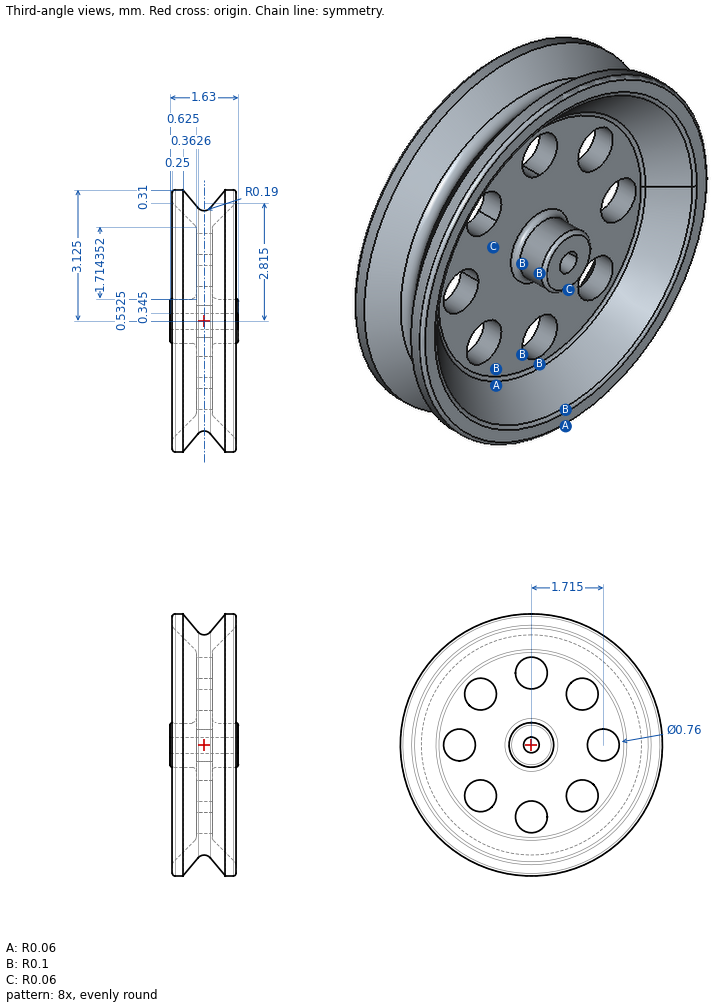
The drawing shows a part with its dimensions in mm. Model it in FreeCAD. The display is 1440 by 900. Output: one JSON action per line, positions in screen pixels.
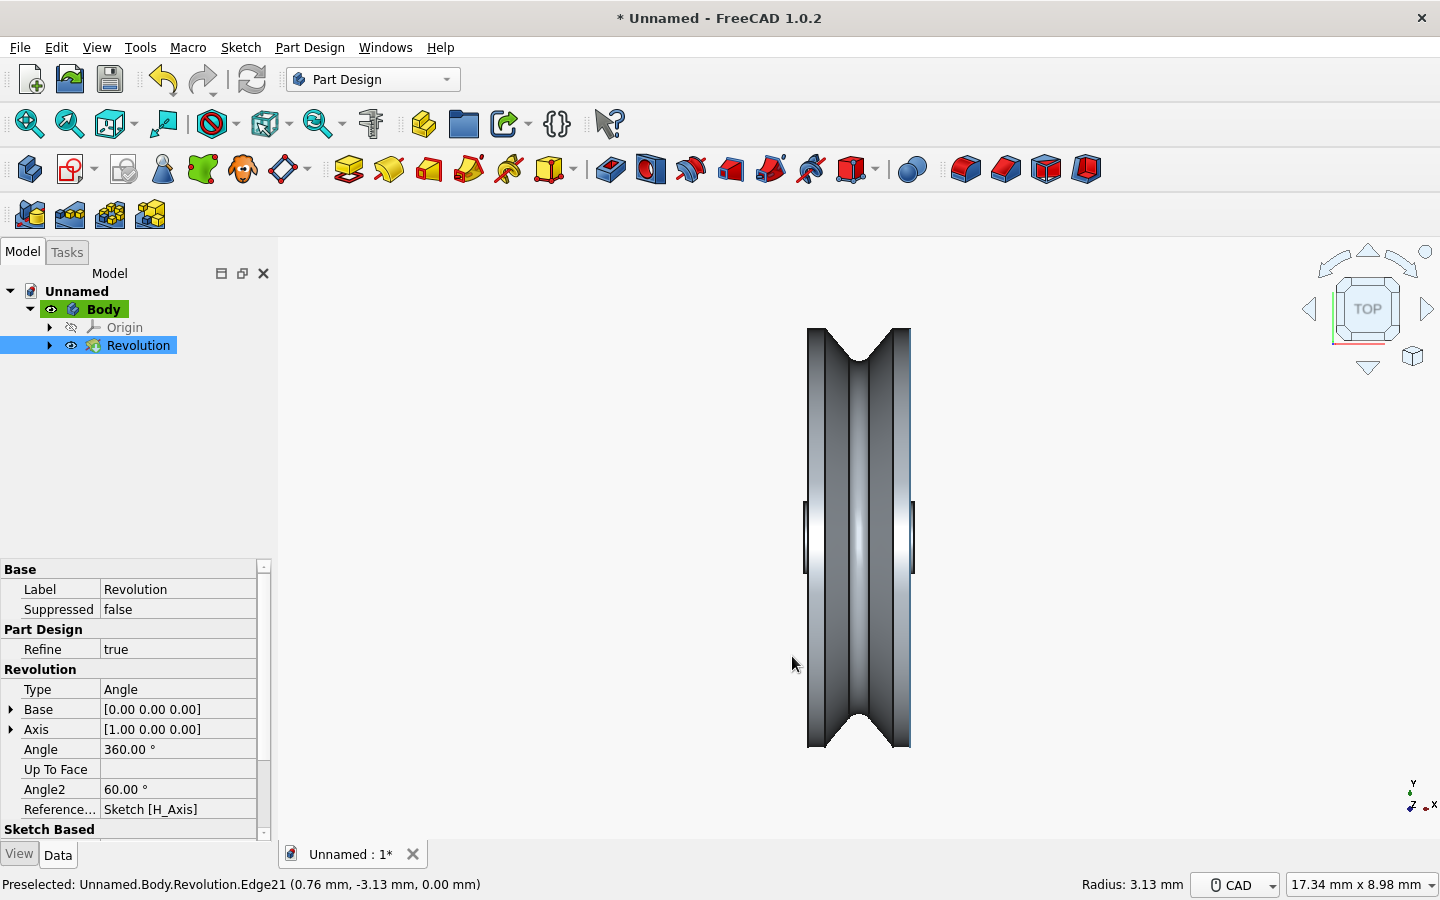
{"action": "left_click", "coordinate": [808, 706], "text": "ctrl"}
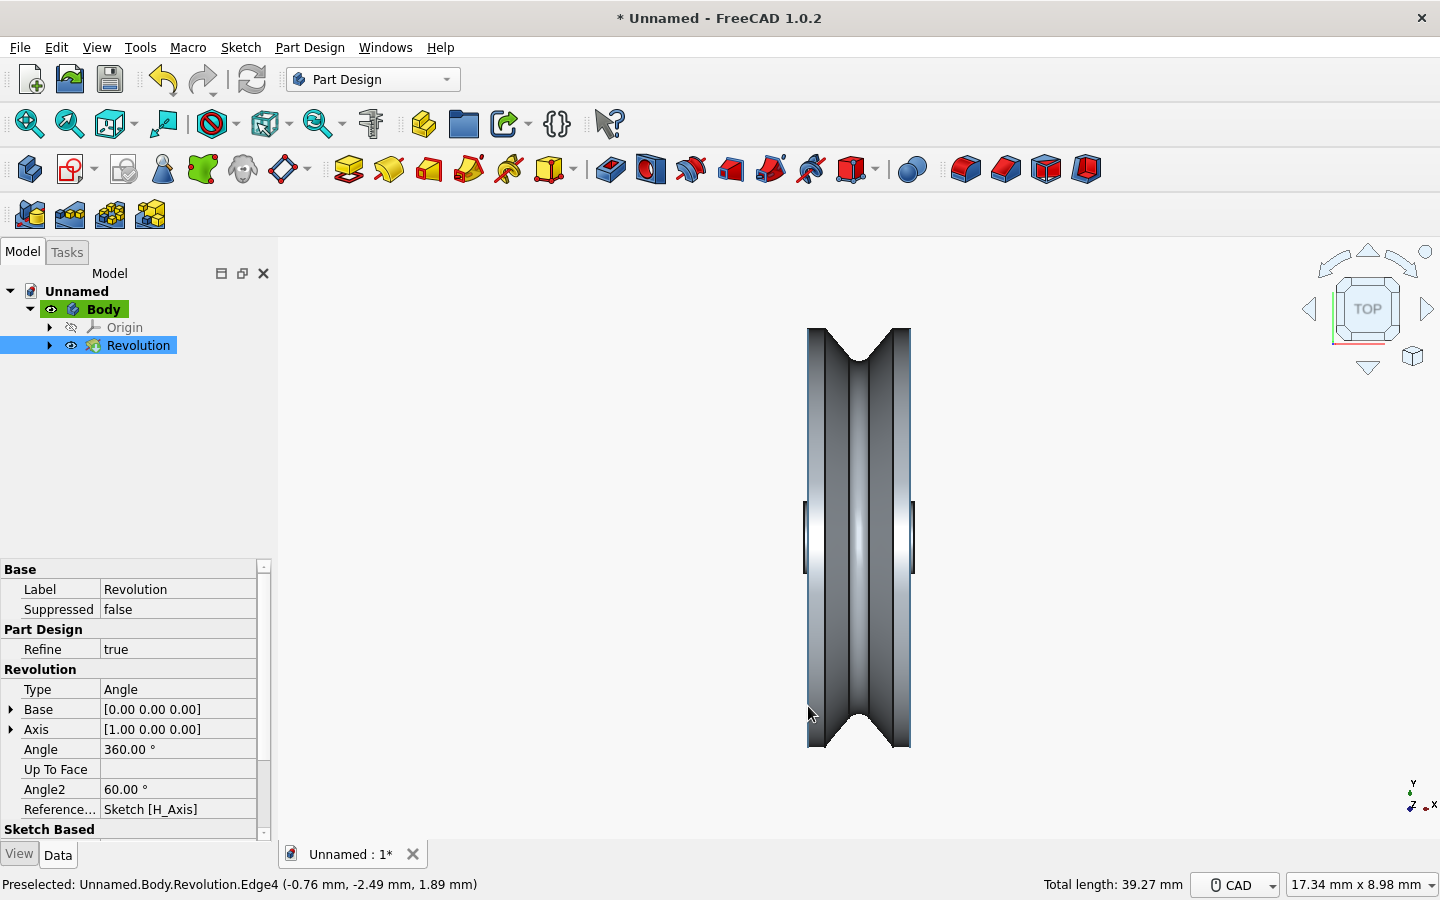
{"action": "left_click", "coordinate": [966, 170]}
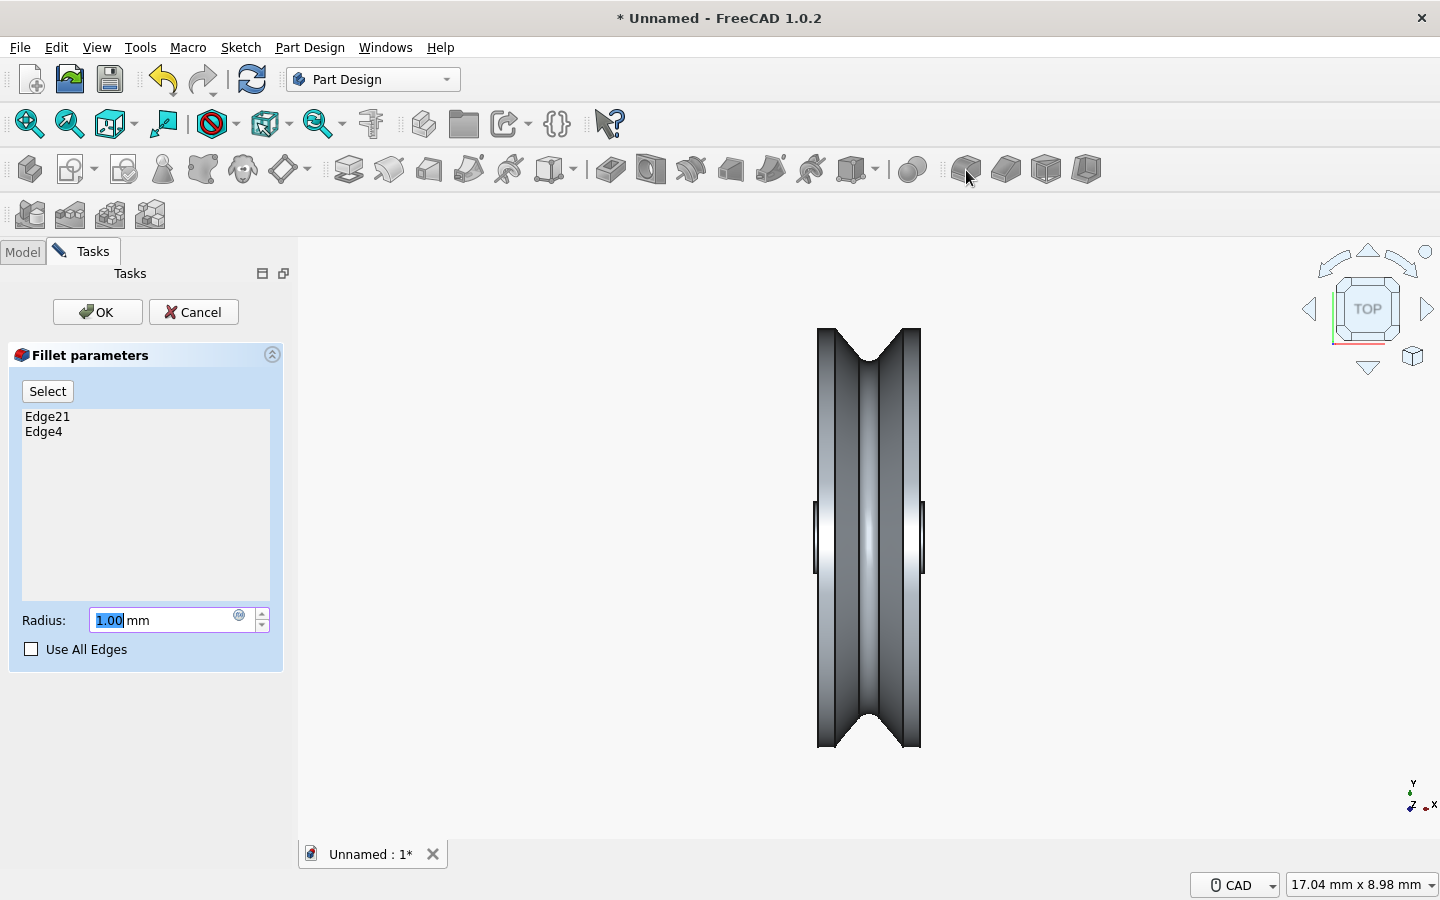
{"action": "type", "text": "0.06"}
{"action": "key", "text": "Tab"}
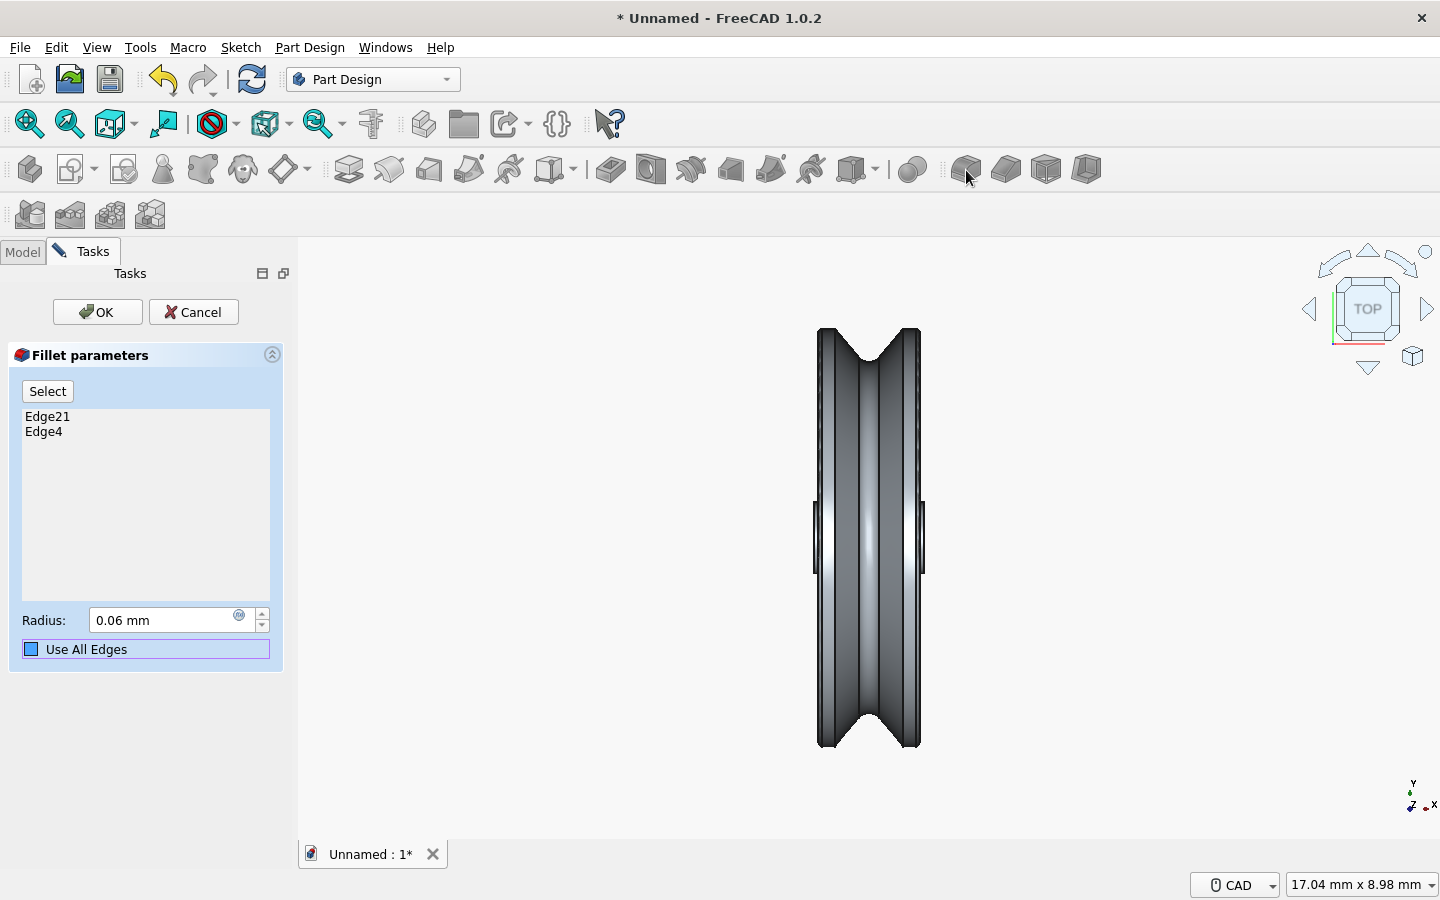
{"action": "left_click", "coordinate": [98, 312]}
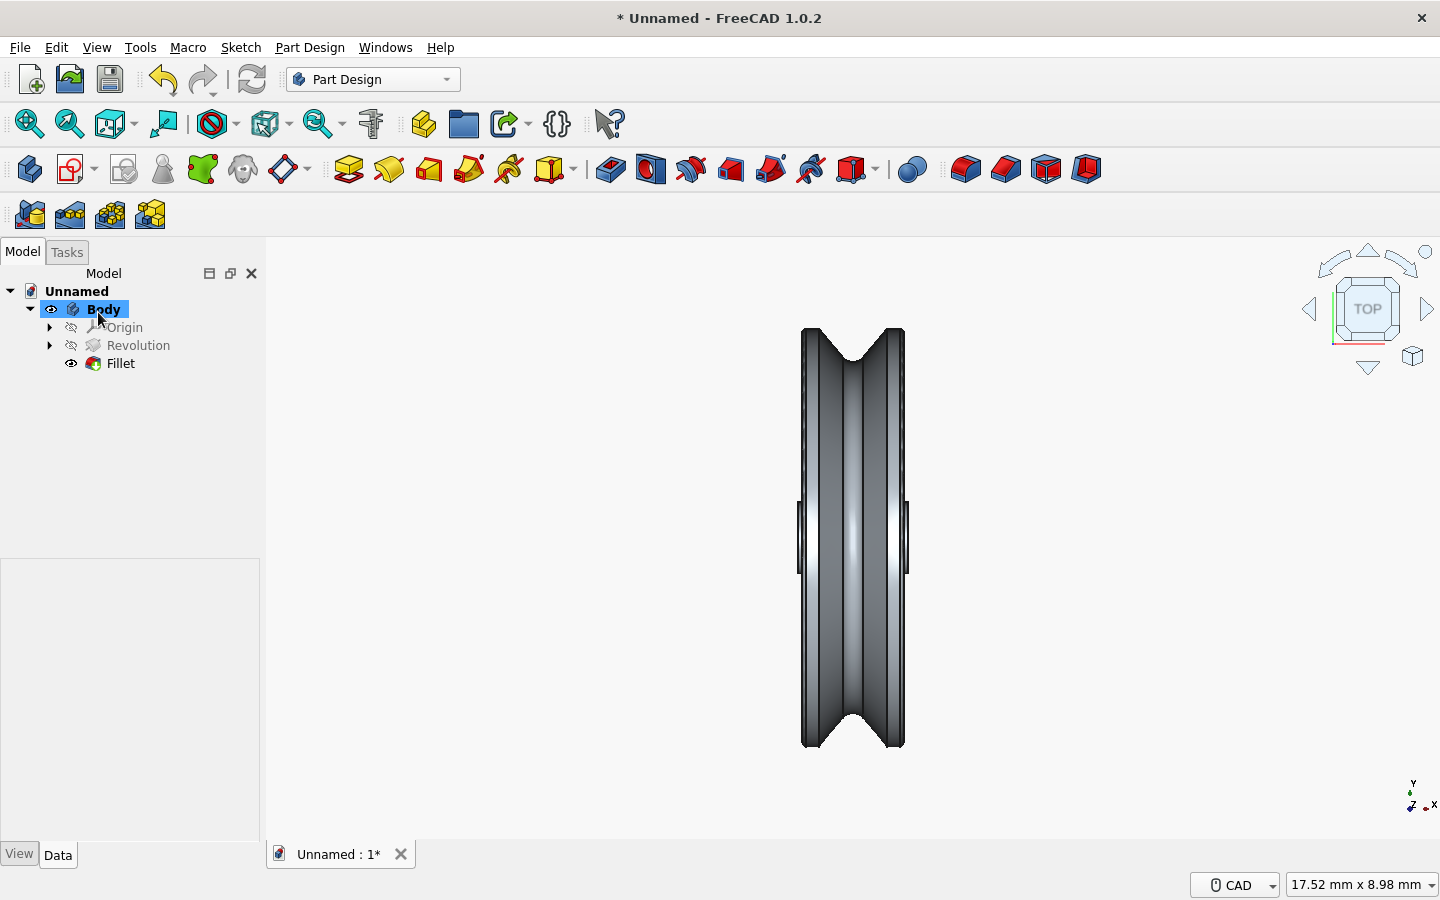
{"action": "key", "text": "0"}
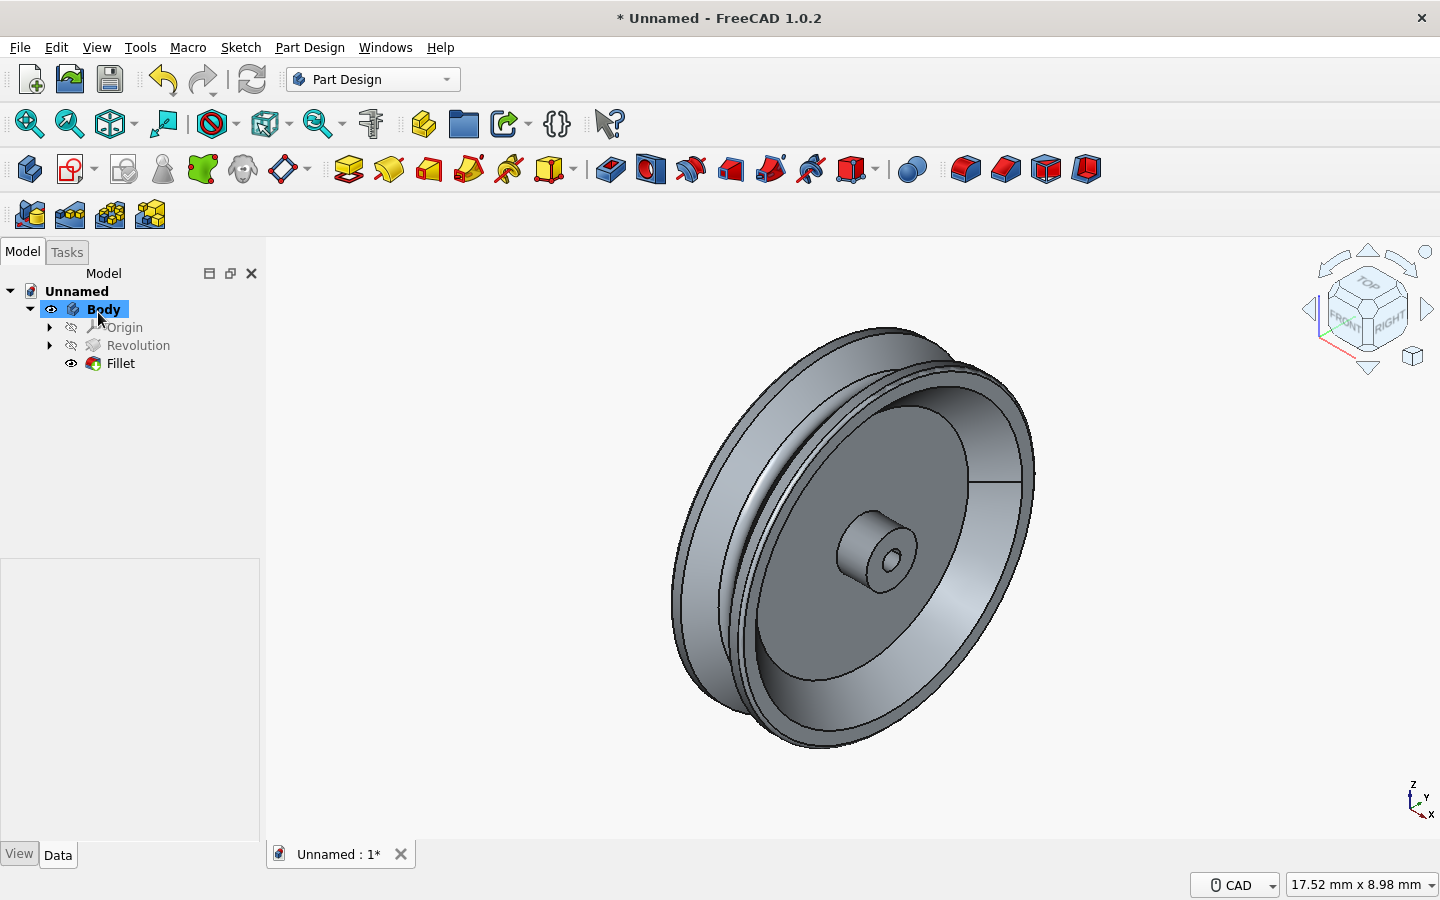
{"action": "left_click", "coordinate": [848, 728]}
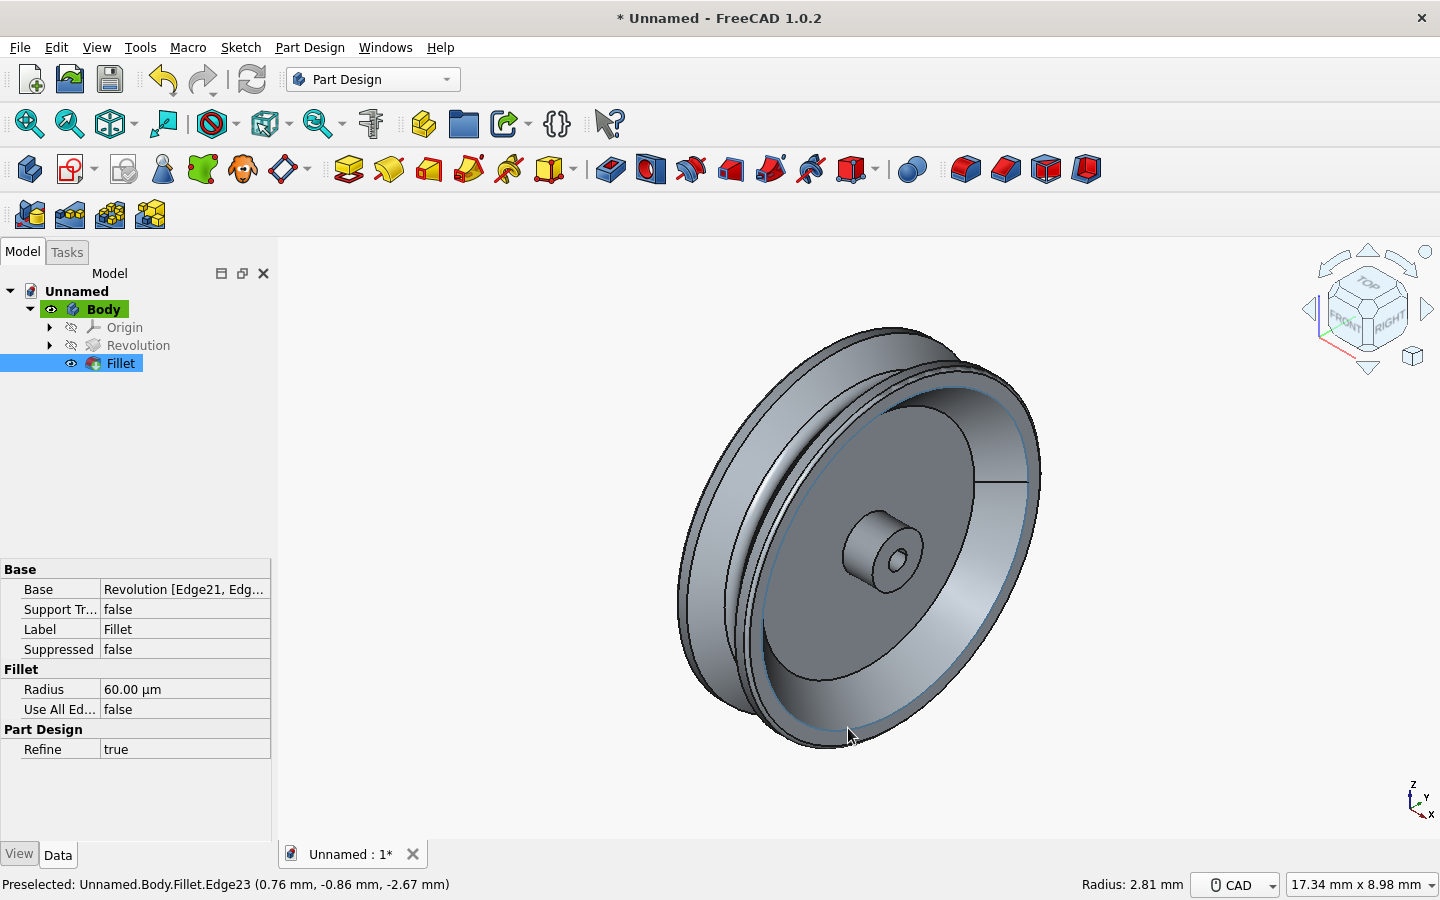
{"action": "key", "text": "2"}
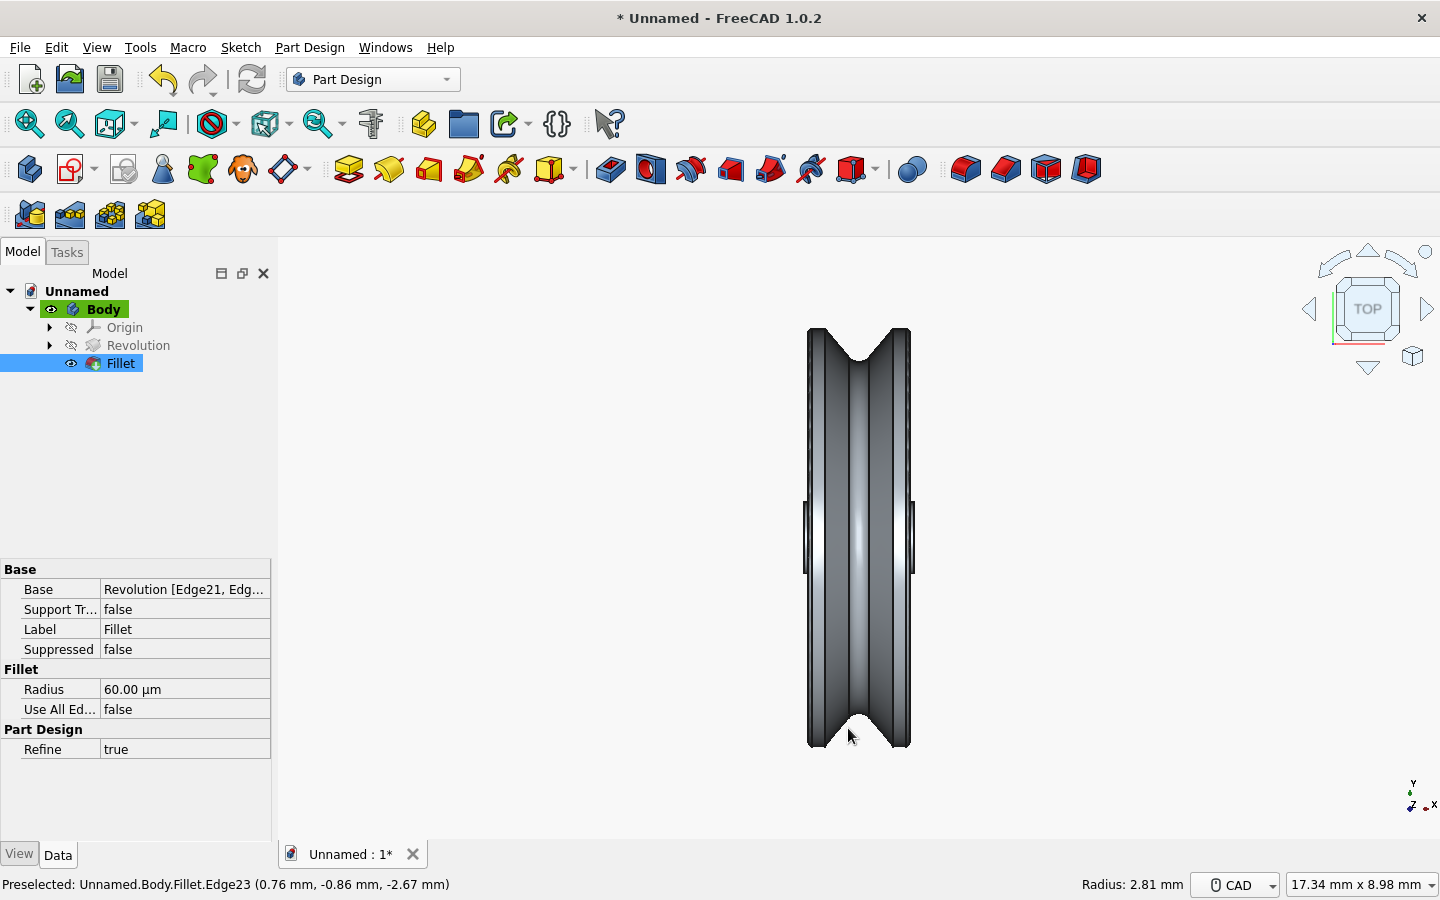
{"action": "key", "text": "1"}